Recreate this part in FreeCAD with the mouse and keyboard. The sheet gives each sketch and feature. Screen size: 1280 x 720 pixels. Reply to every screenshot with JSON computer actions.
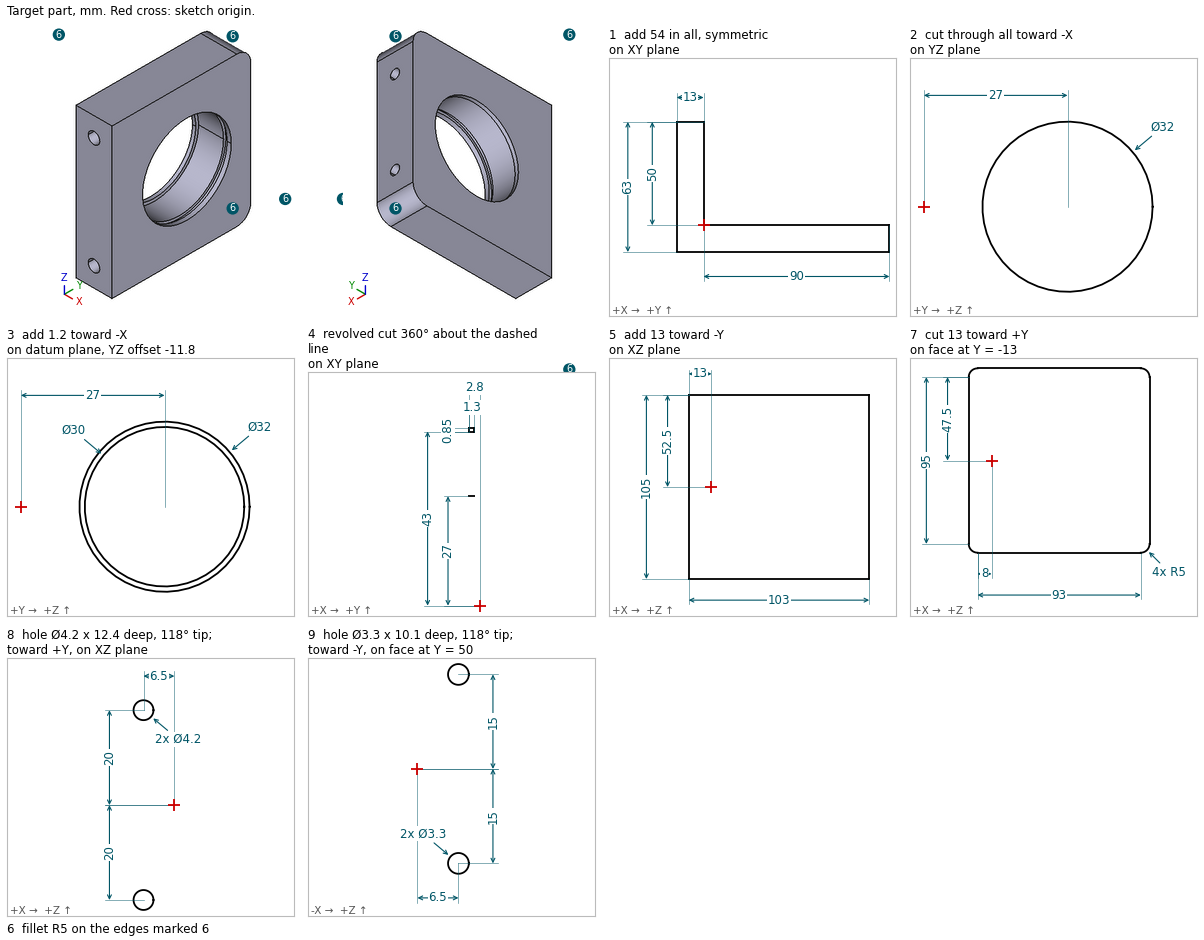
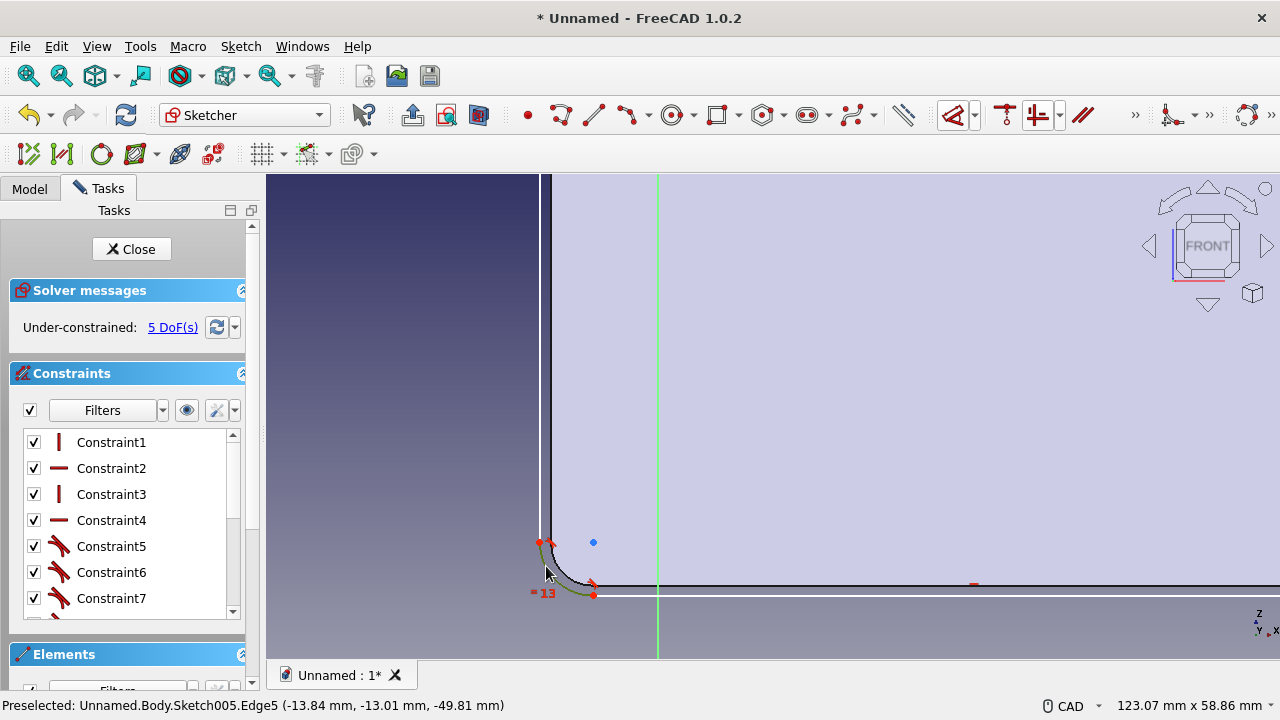
{"action": "key", "text": "k r"}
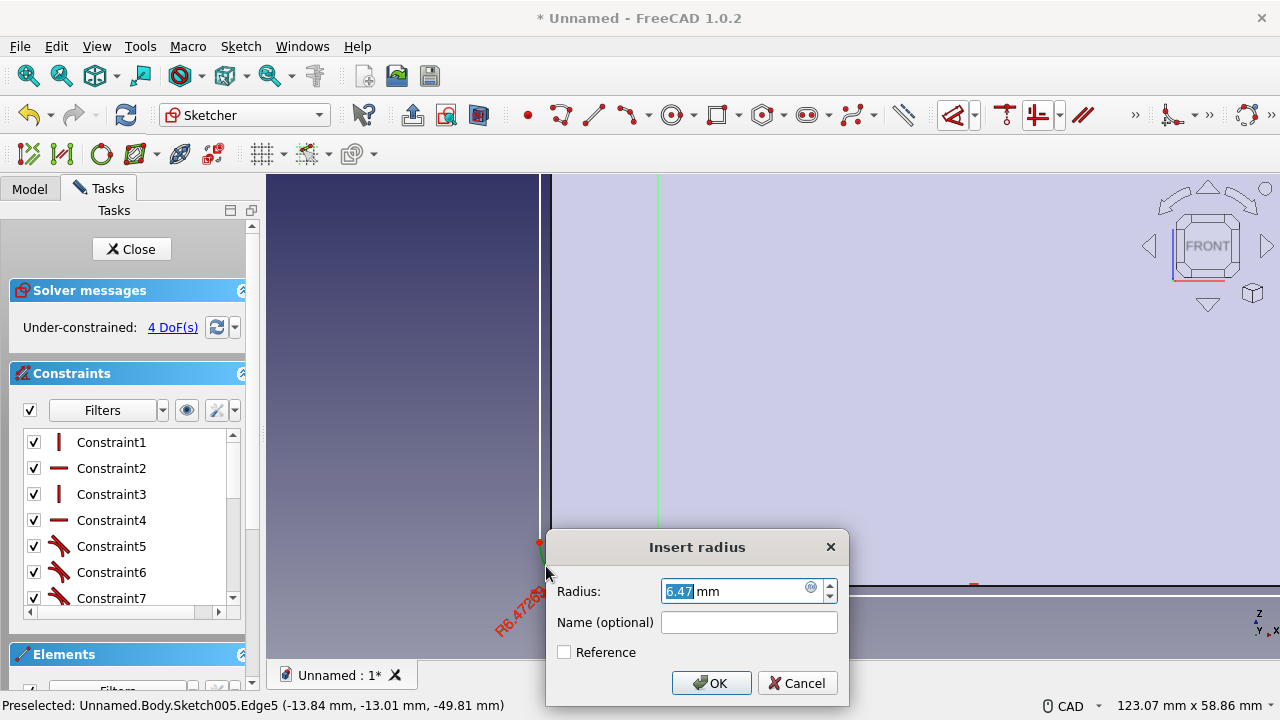
{"action": "type", "text": "5"}
{"action": "key", "text": "Return"}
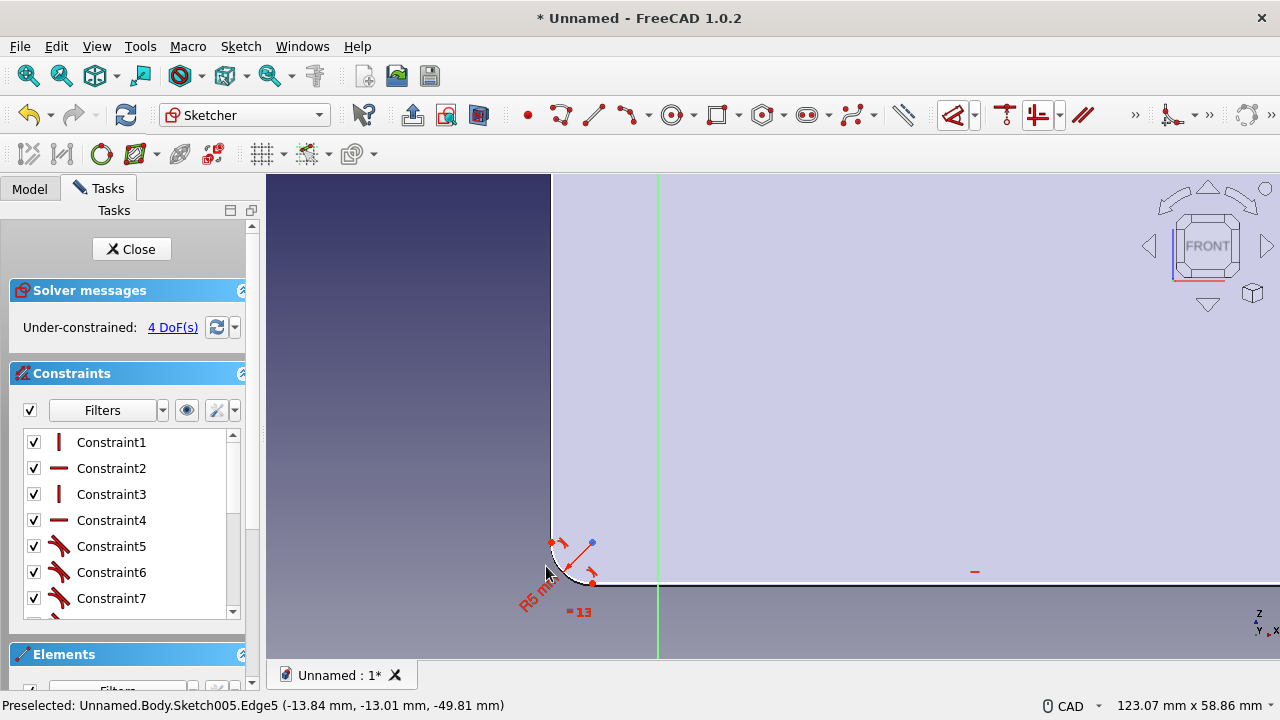
{"action": "left_click", "coordinate": [552, 310]}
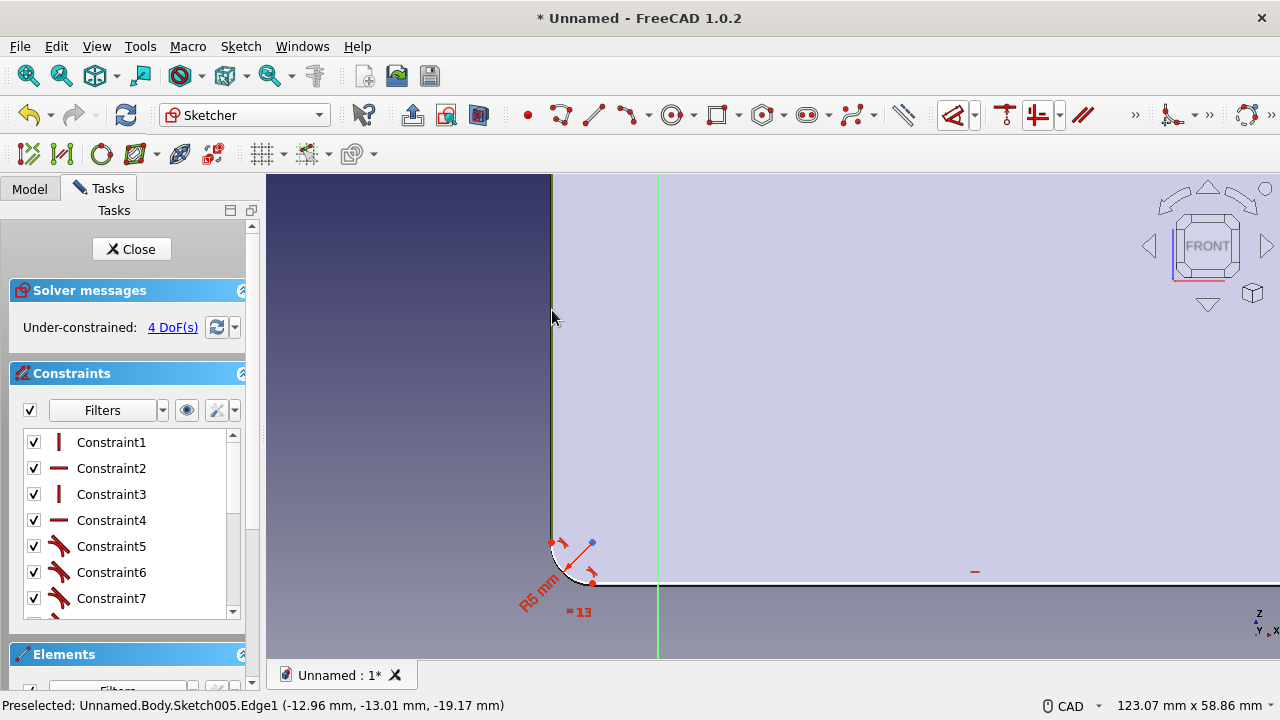
{"action": "left_click", "coordinate": [974, 116]}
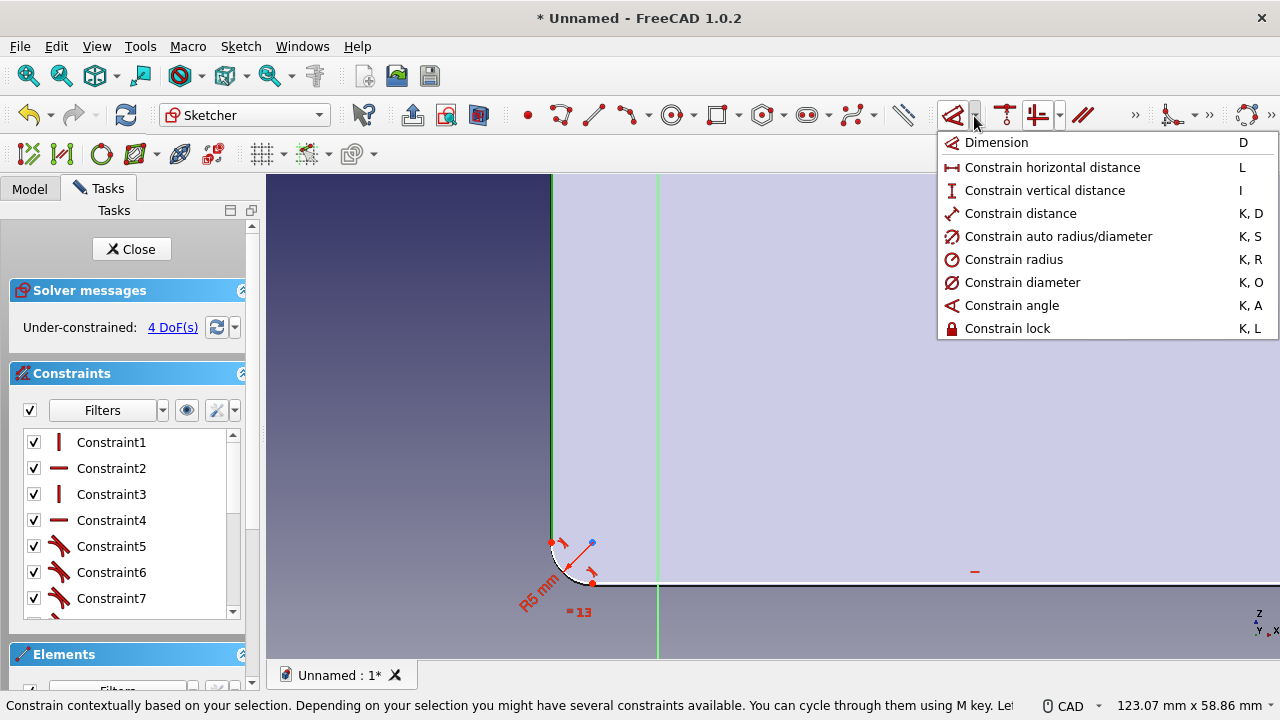
{"action": "left_click", "coordinate": [1108, 190]}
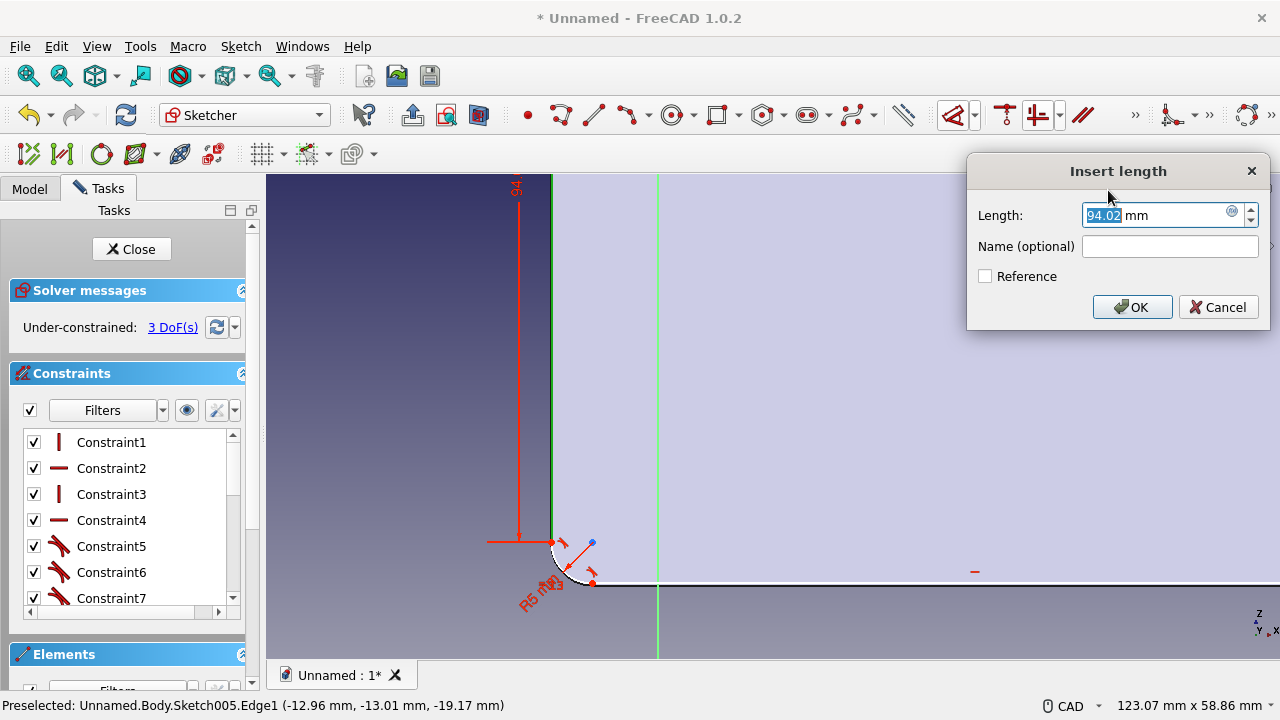
{"action": "type", "text": "95"}
{"action": "key", "text": "Return"}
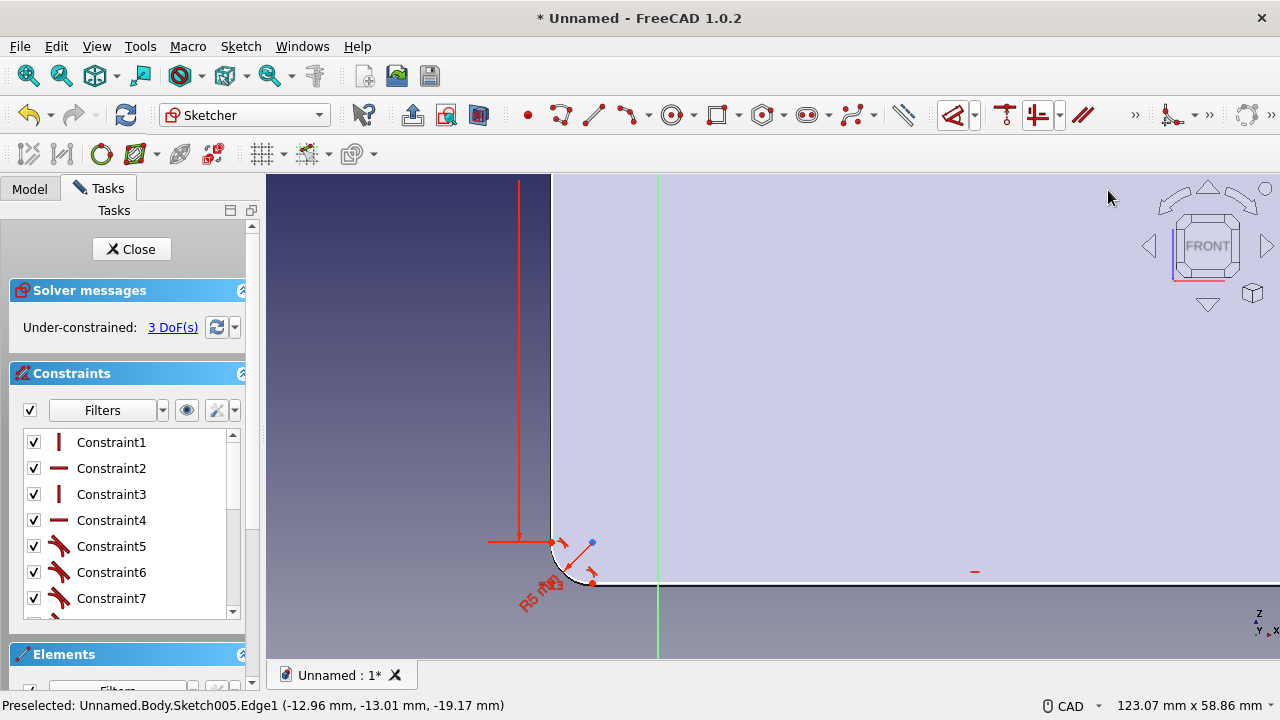
{"action": "left_click", "coordinate": [823, 583]}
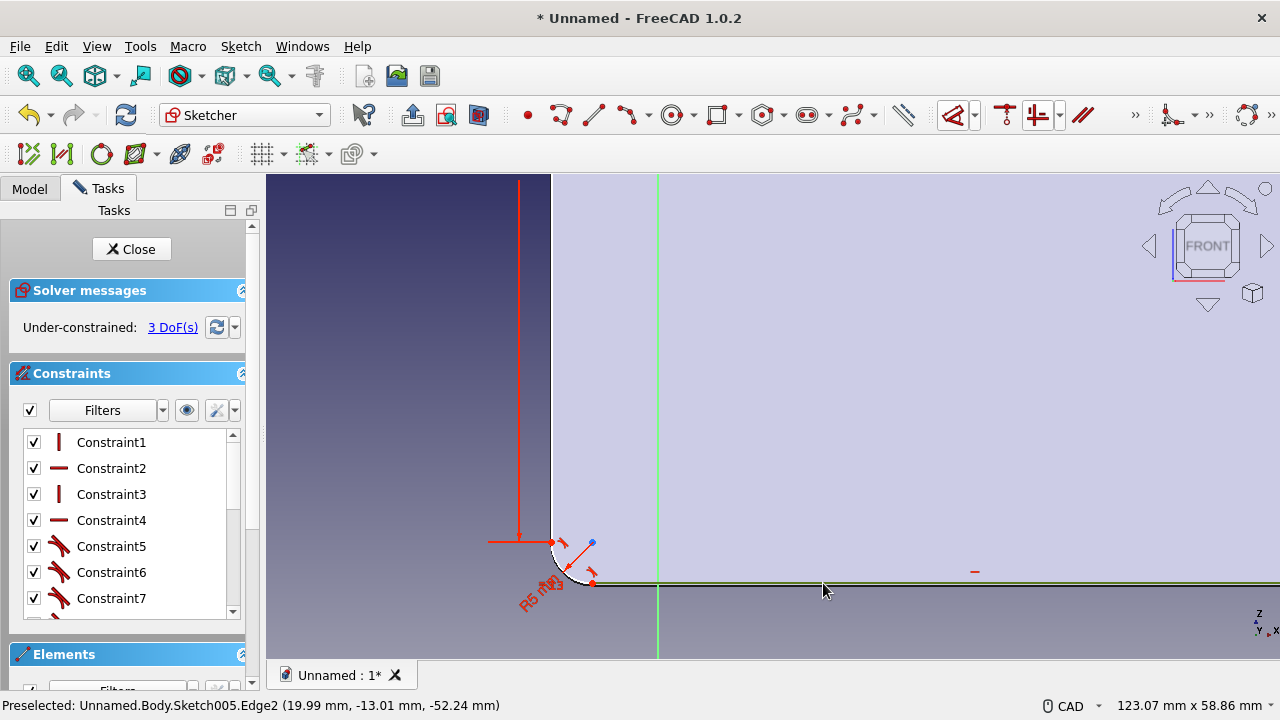
{"action": "key", "text": "l"}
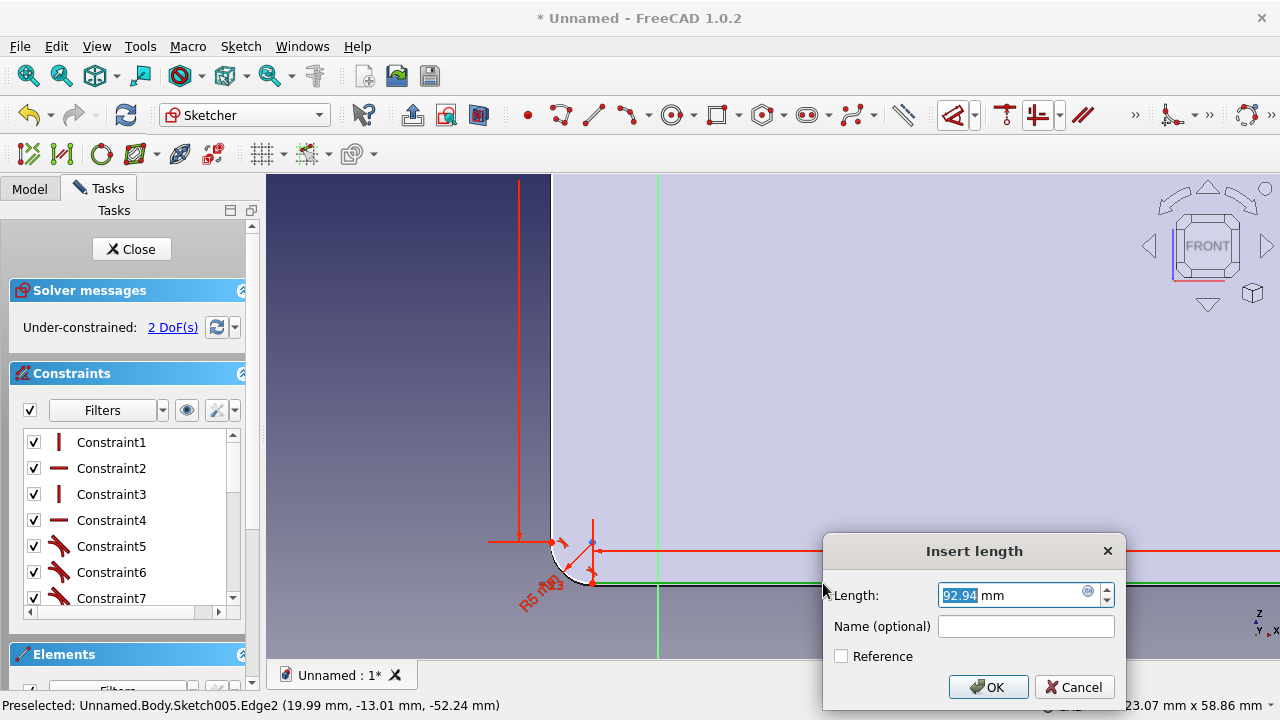
{"action": "type", "text": "93"}
{"action": "key", "text": "Return"}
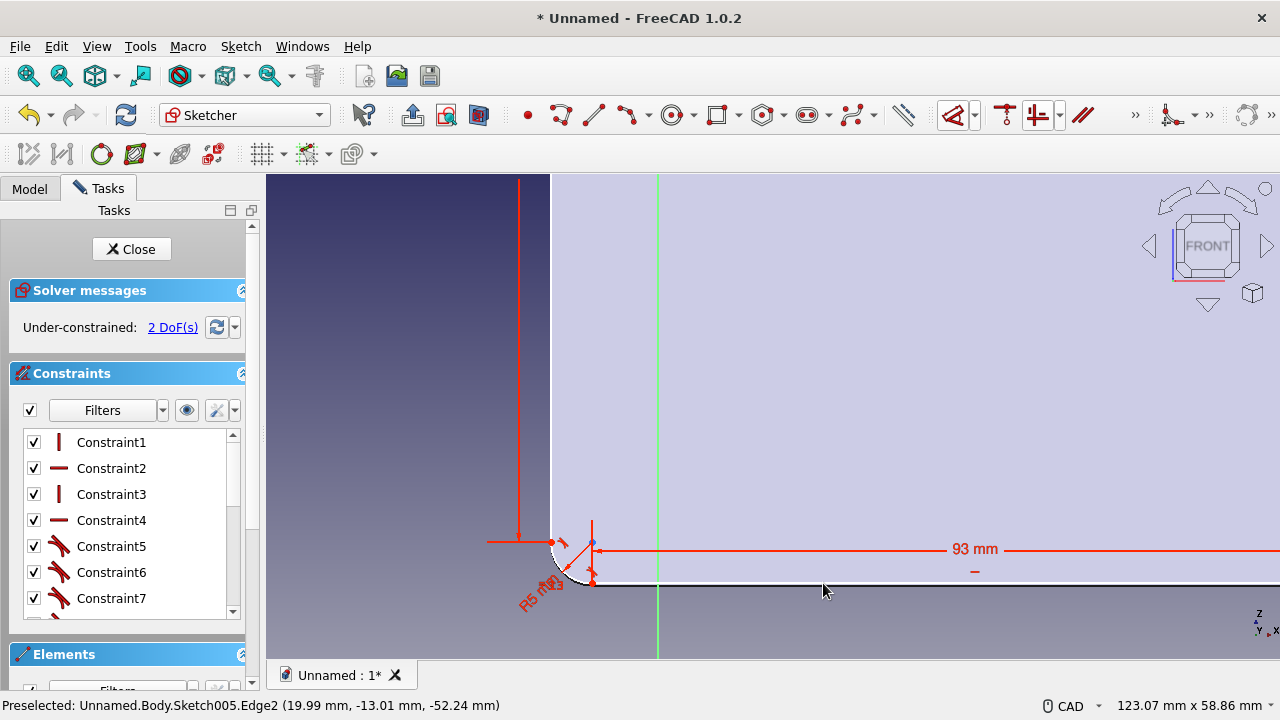
{"action": "left_click", "coordinate": [592, 583]}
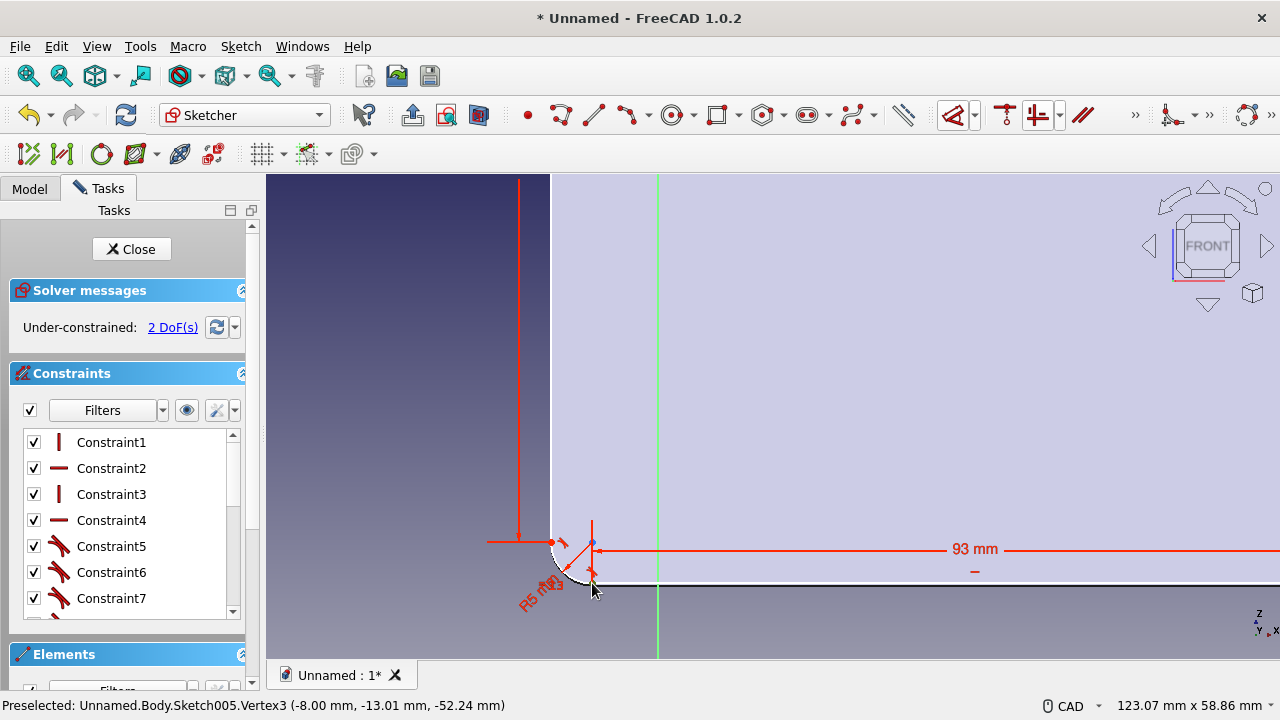
{"action": "key", "text": "l"}